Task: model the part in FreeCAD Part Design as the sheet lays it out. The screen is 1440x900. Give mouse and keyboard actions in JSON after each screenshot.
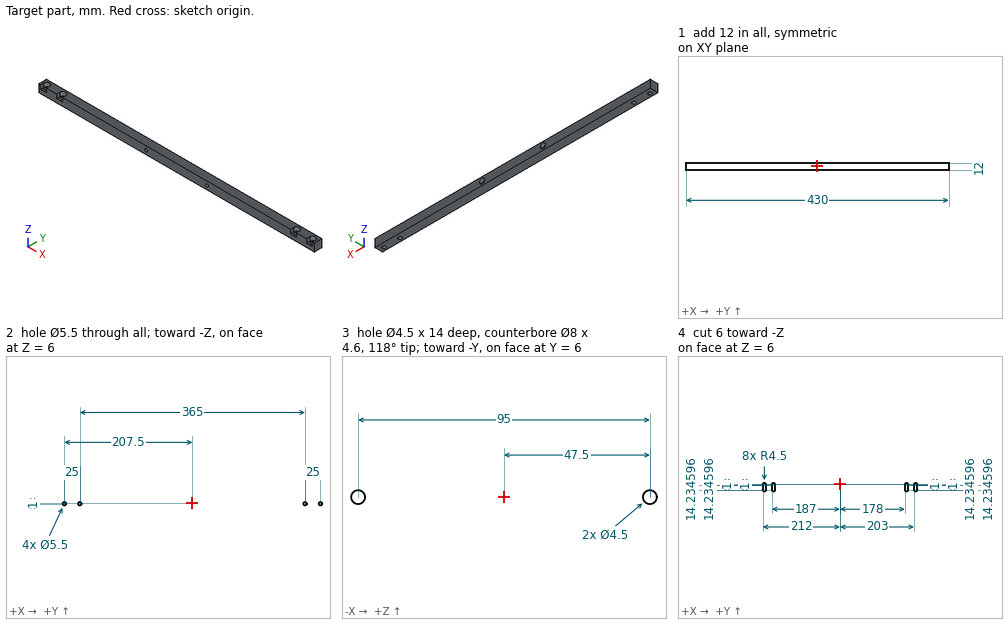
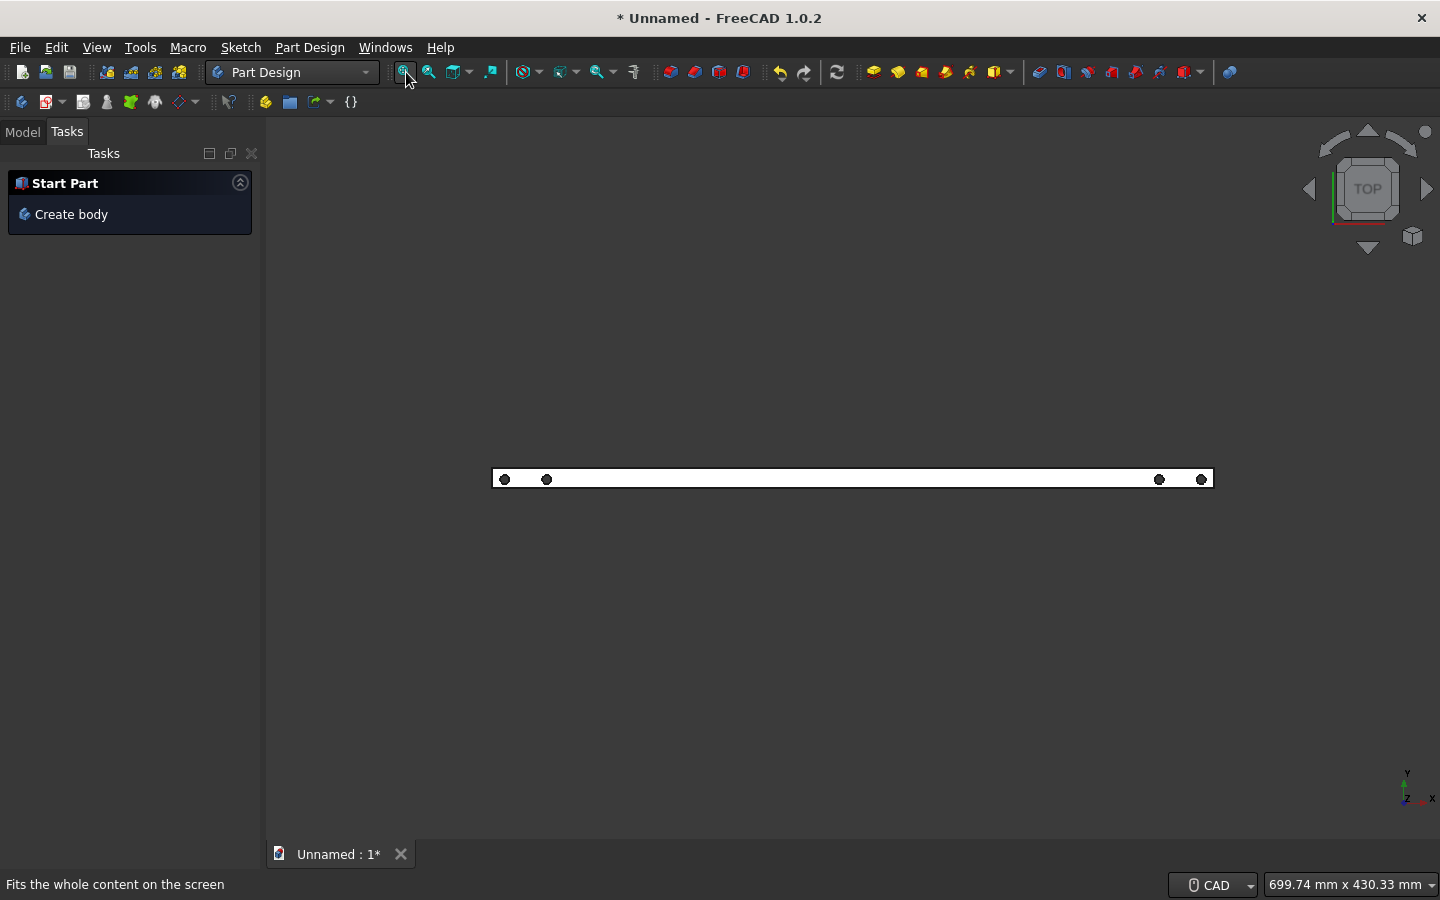
{"action": "left_click", "coordinate": [1059, 477]}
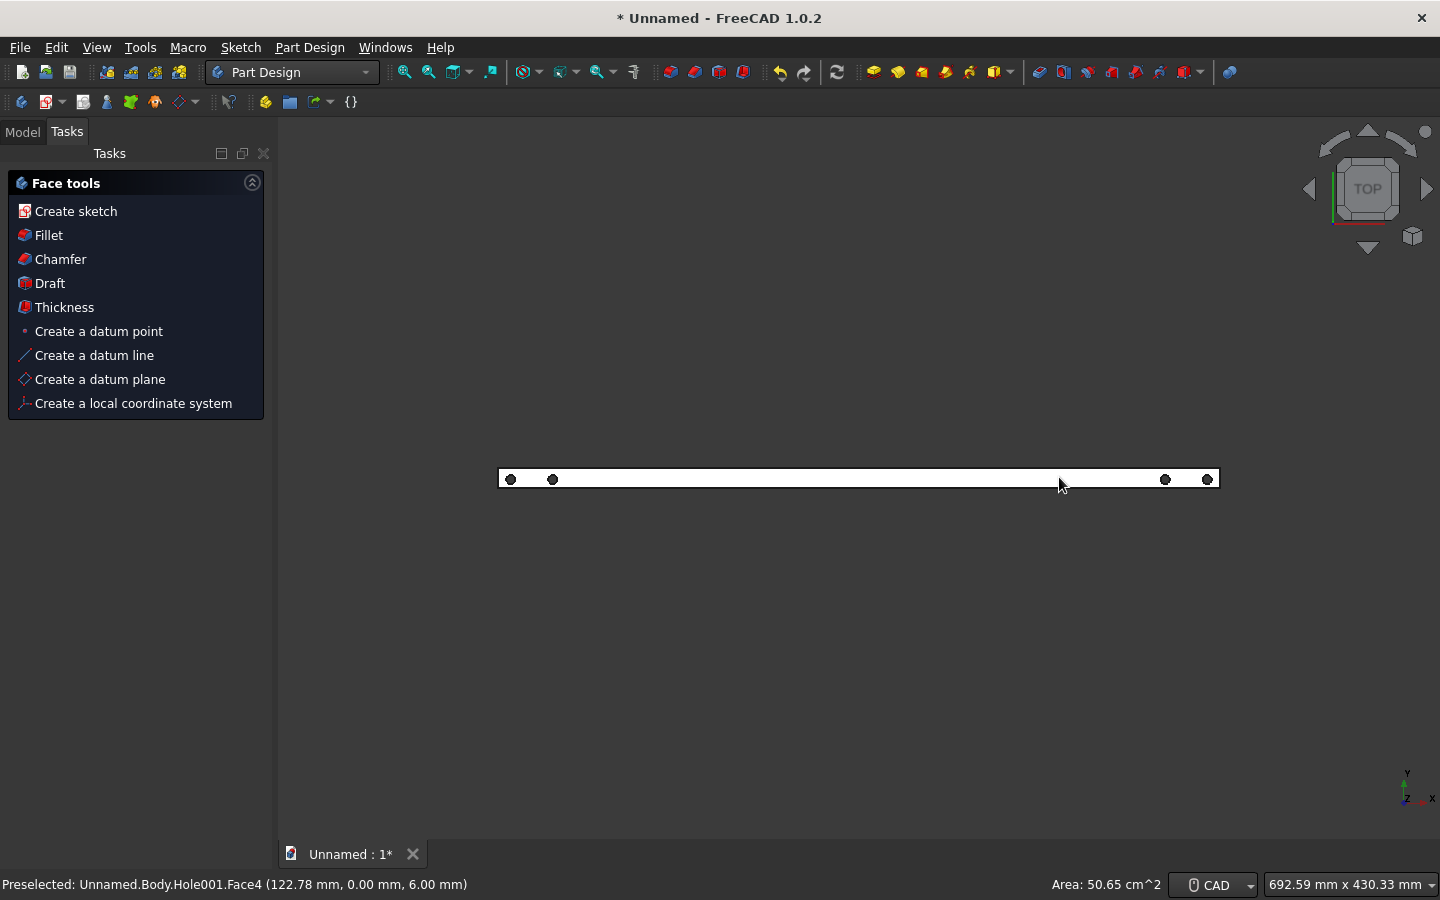
{"action": "left_click", "coordinate": [46, 102]}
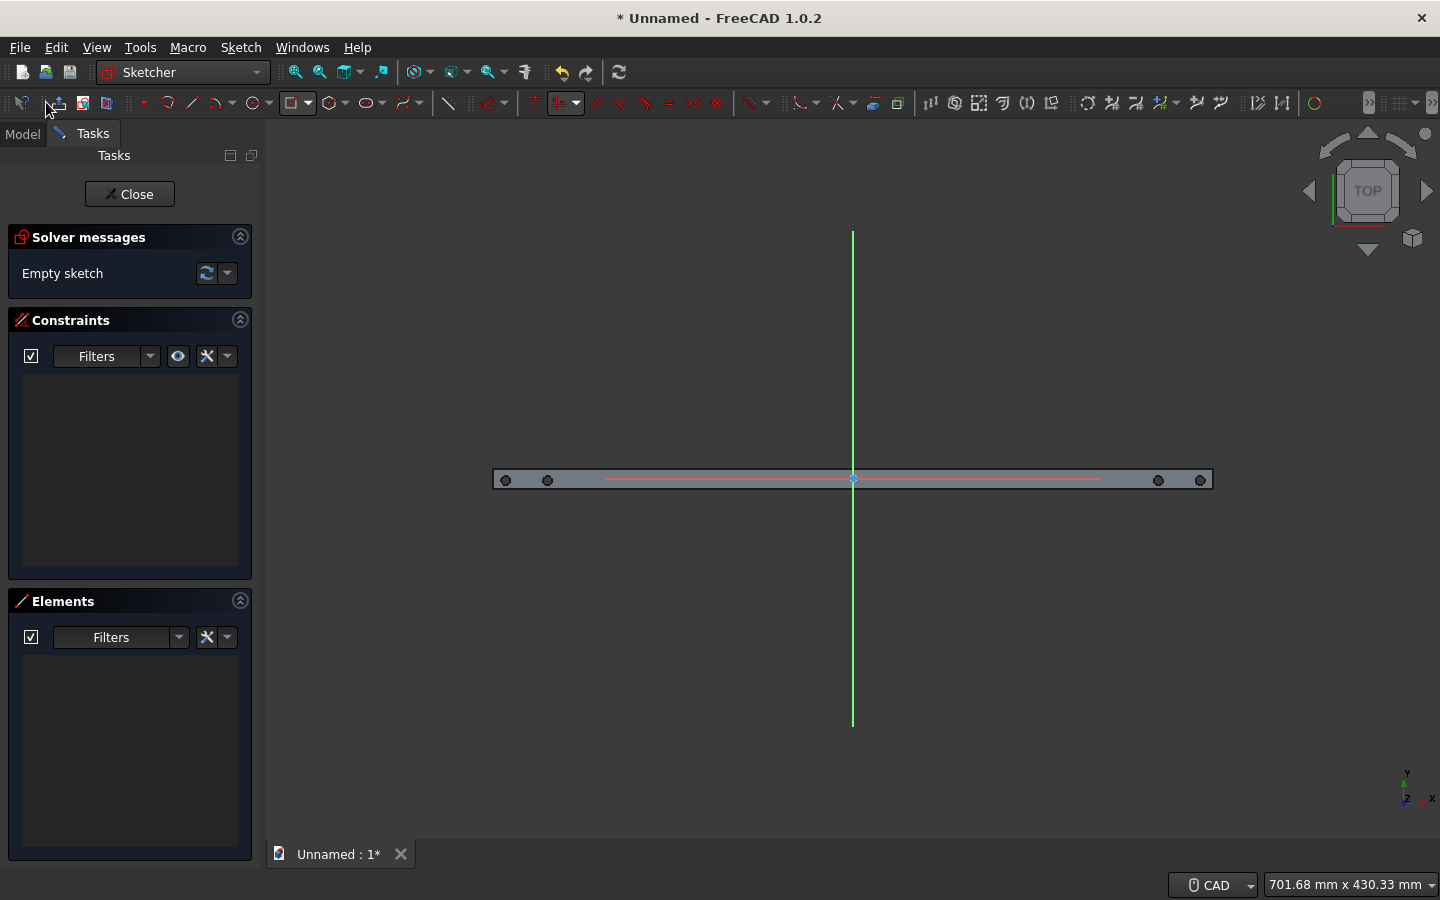
{"action": "left_click", "coordinate": [366, 104]}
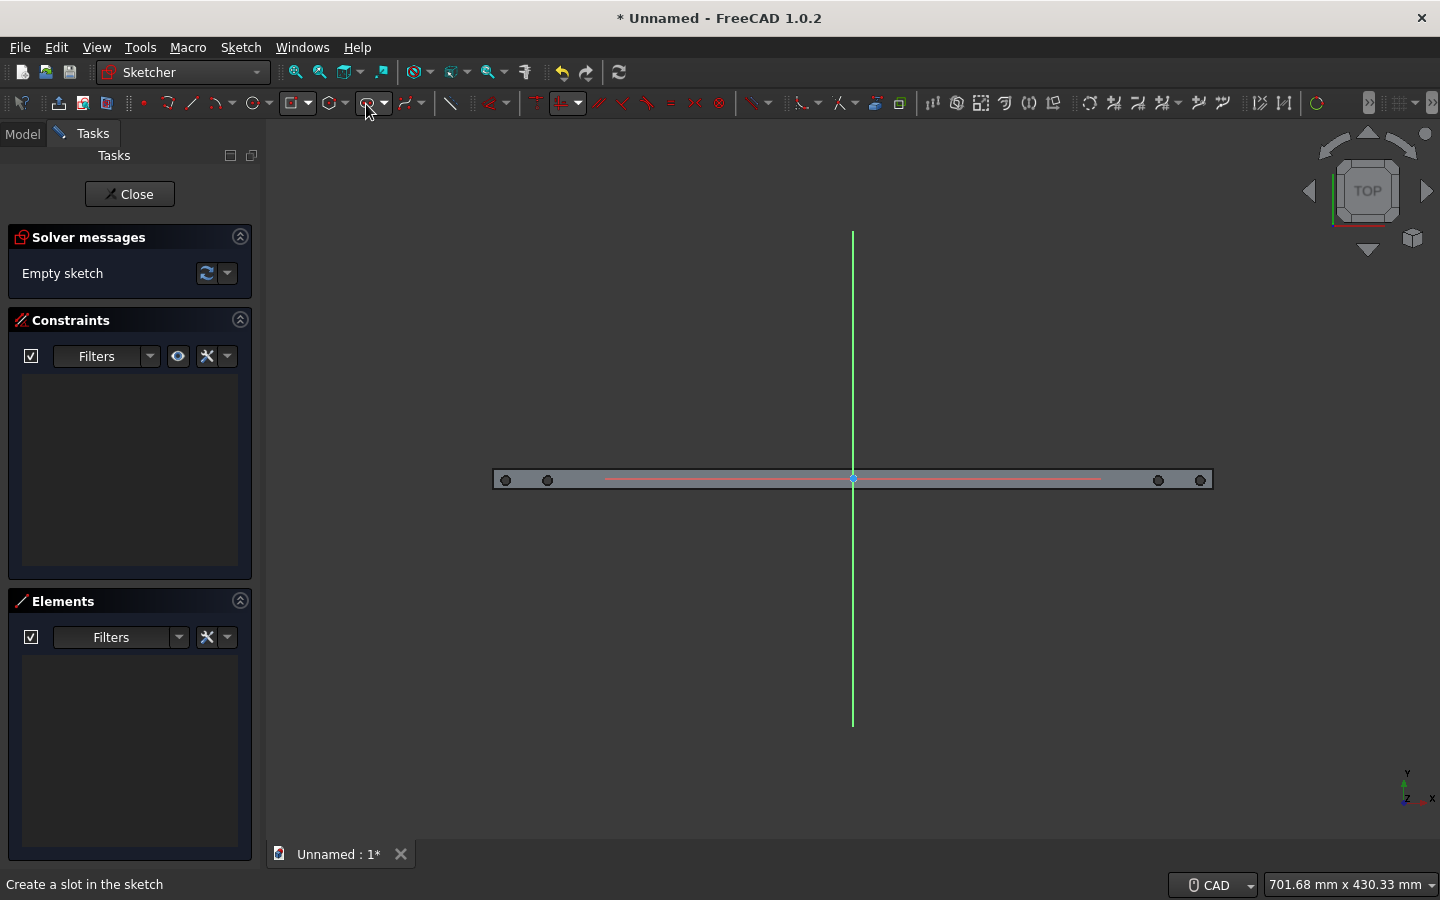
{"action": "scroll", "coordinate": [506, 504], "scroll_direction": "up", "scroll_amount": 6}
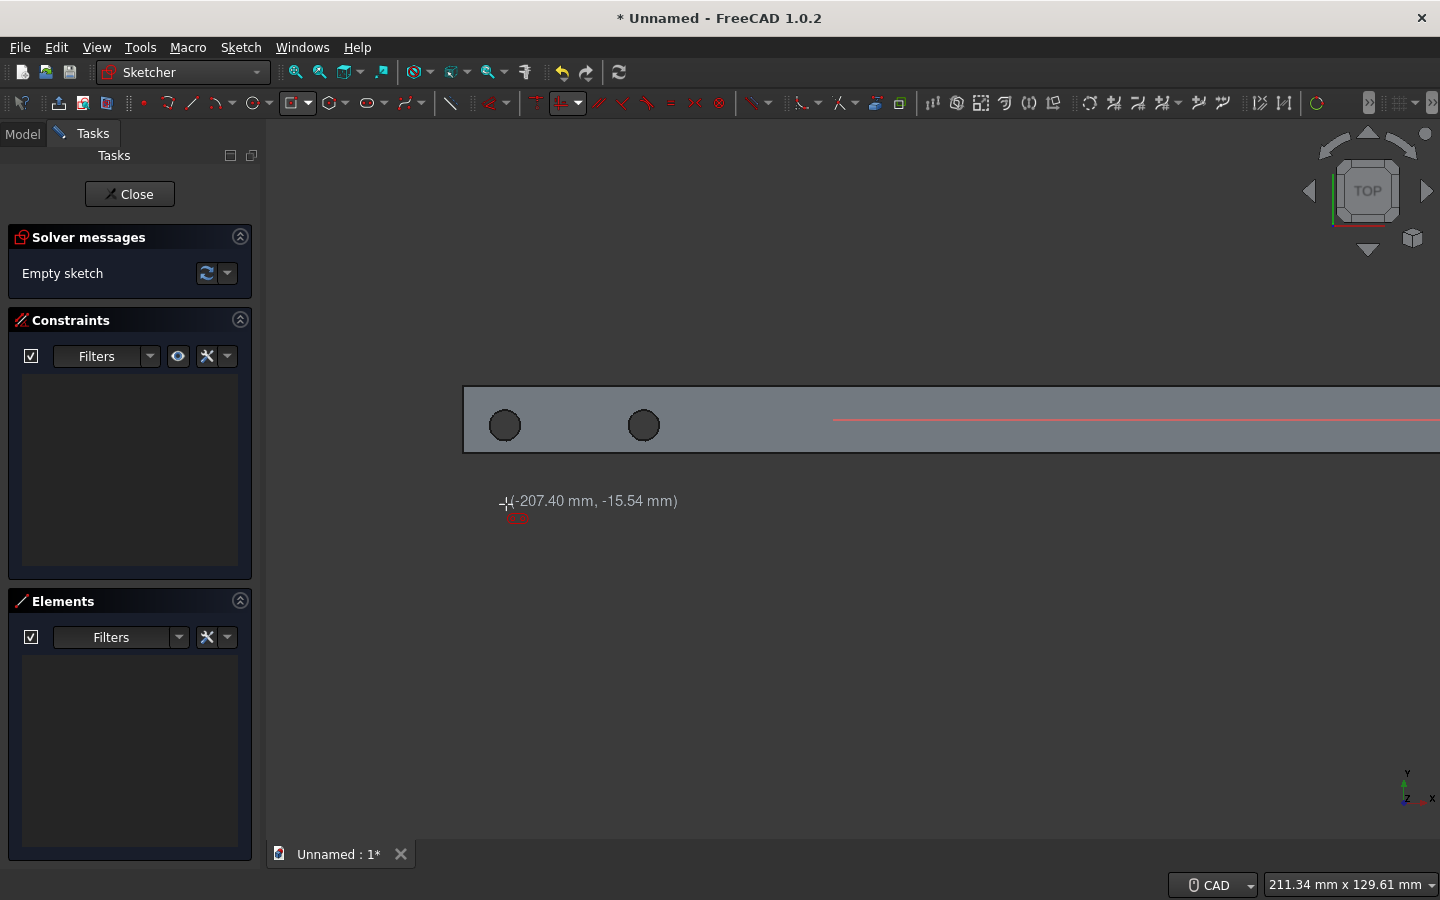
{"action": "left_click", "coordinate": [505, 504]}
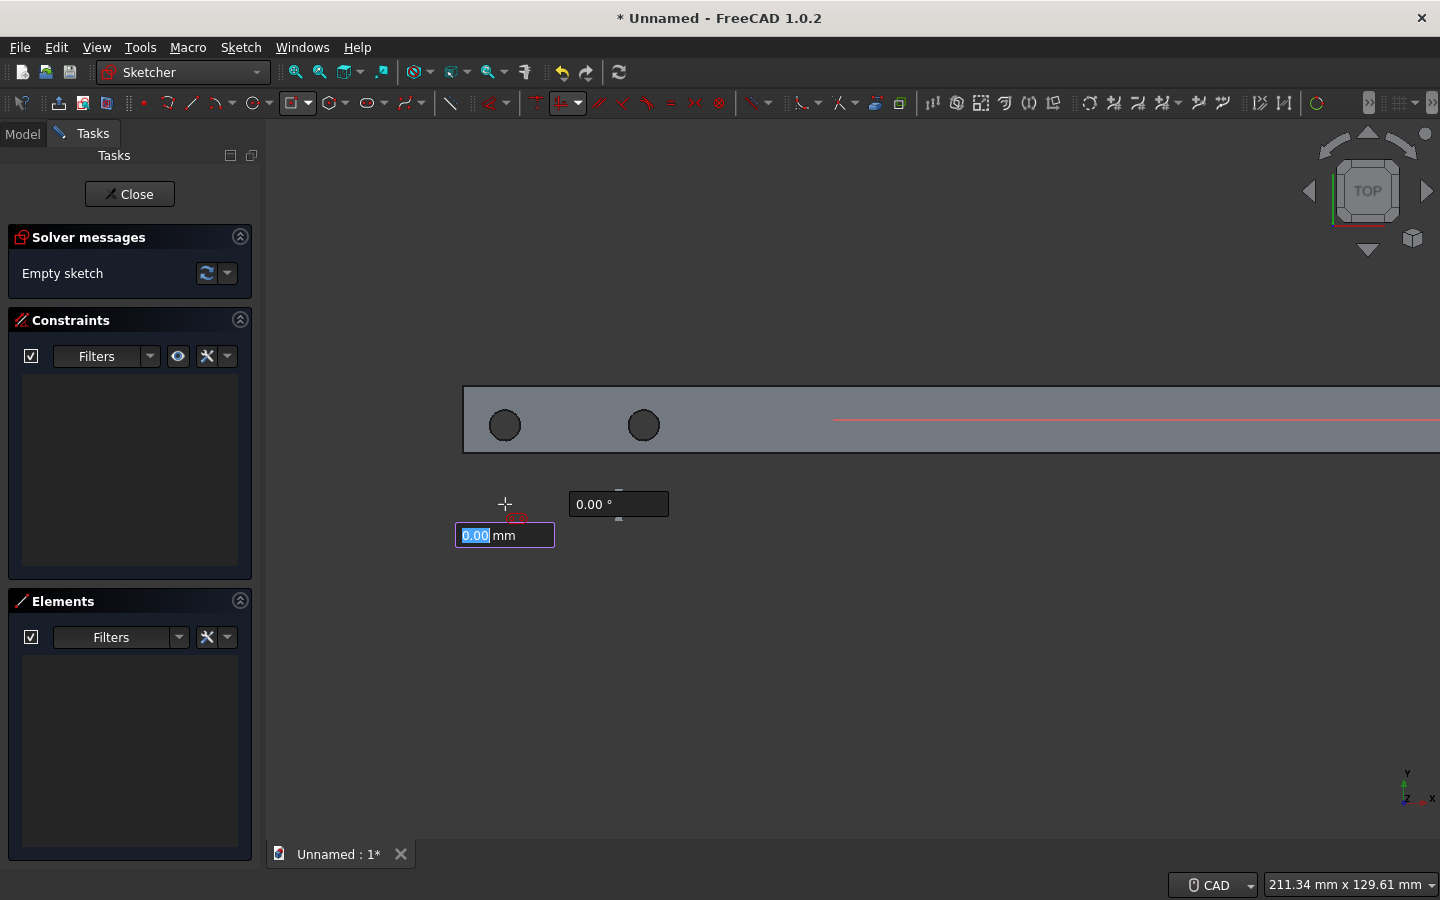
{"action": "scroll", "coordinate": [505, 425], "scroll_direction": "up", "scroll_amount": 6}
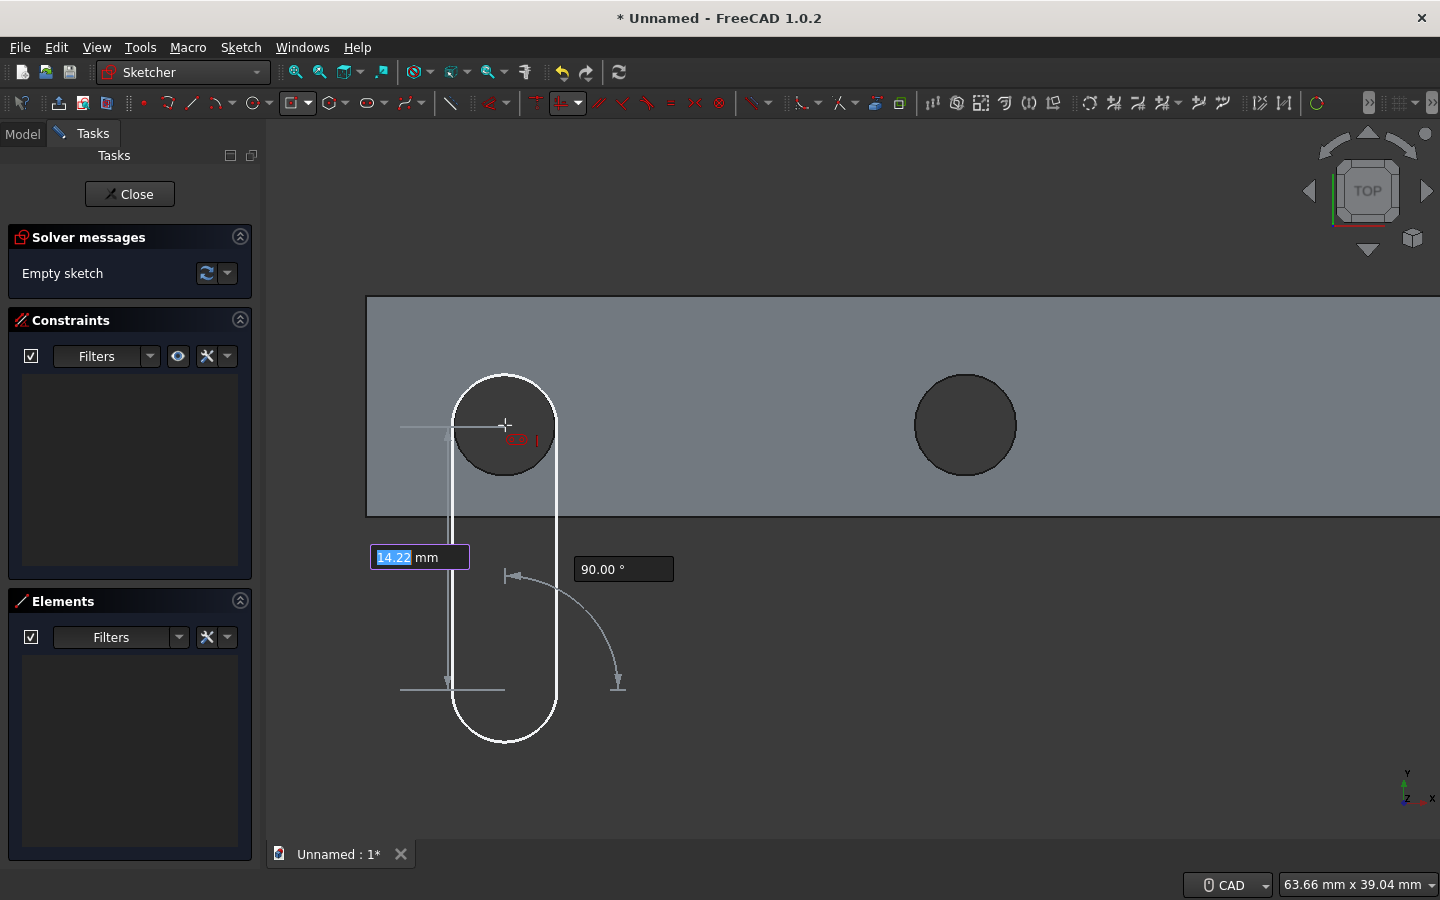
{"action": "left_click", "coordinate": [505, 425]}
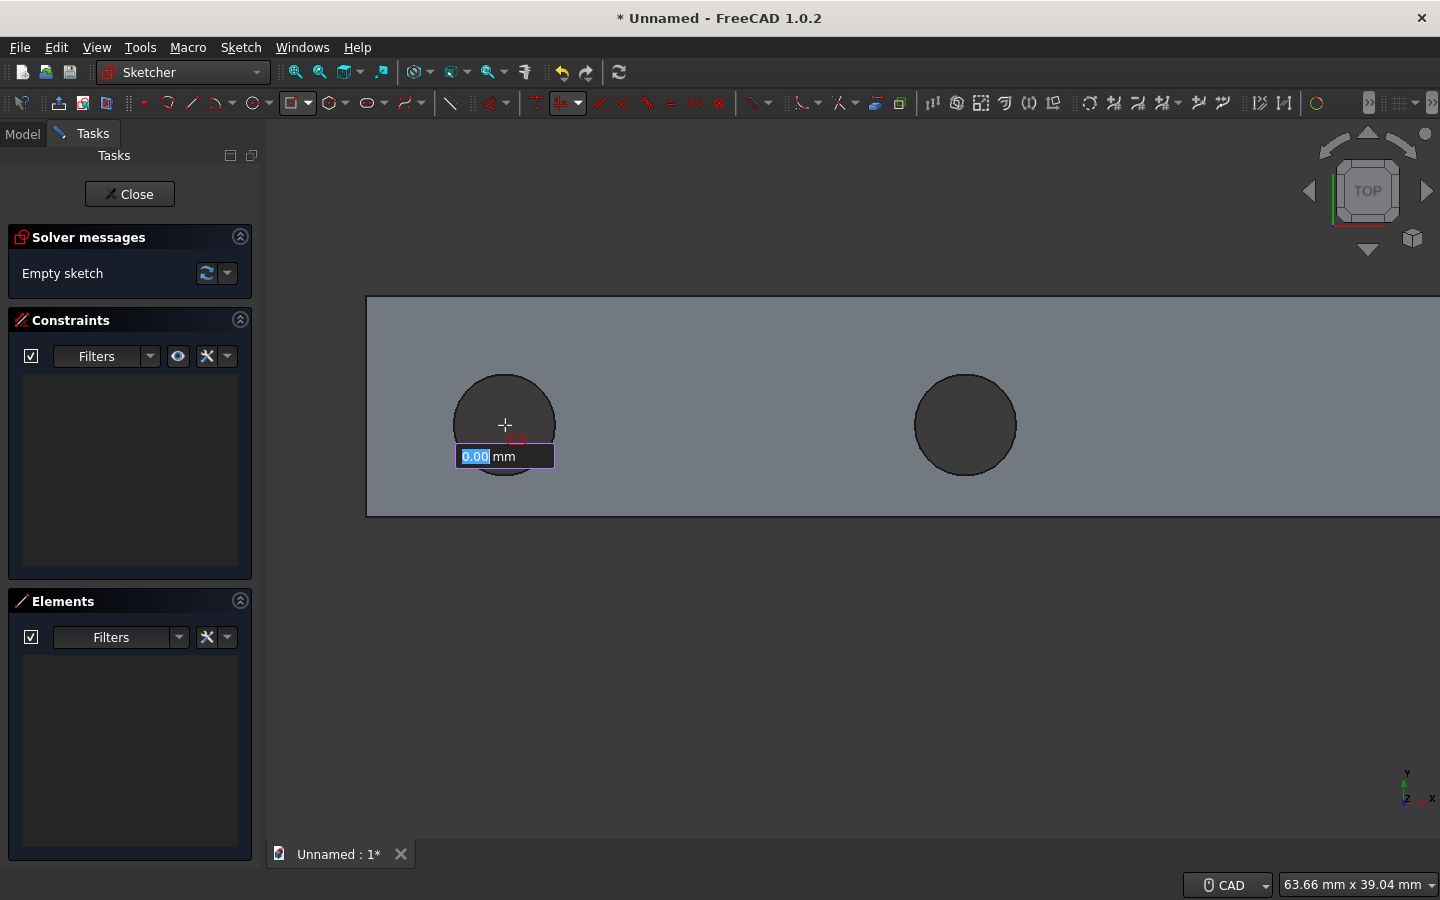
{"action": "scroll", "coordinate": [431, 471], "scroll_direction": "down", "scroll_amount": 12}